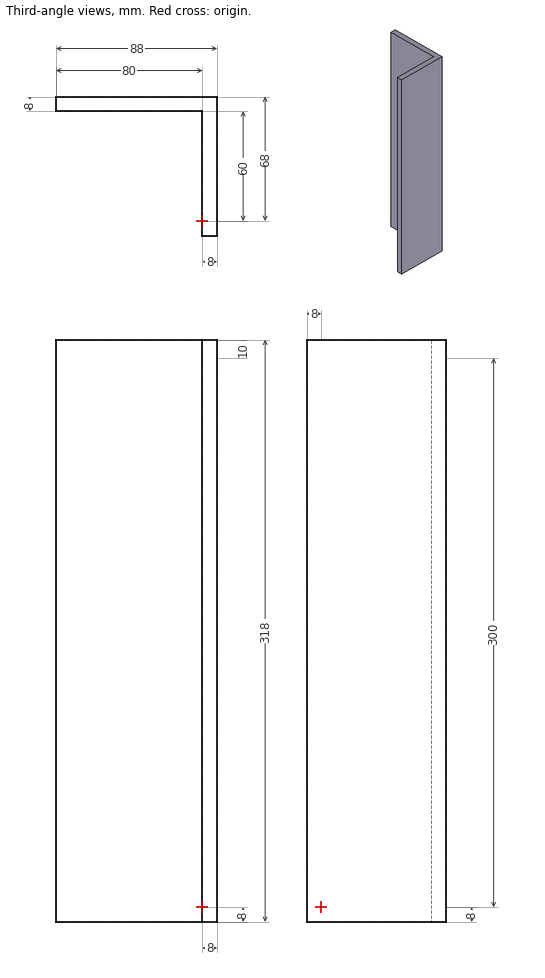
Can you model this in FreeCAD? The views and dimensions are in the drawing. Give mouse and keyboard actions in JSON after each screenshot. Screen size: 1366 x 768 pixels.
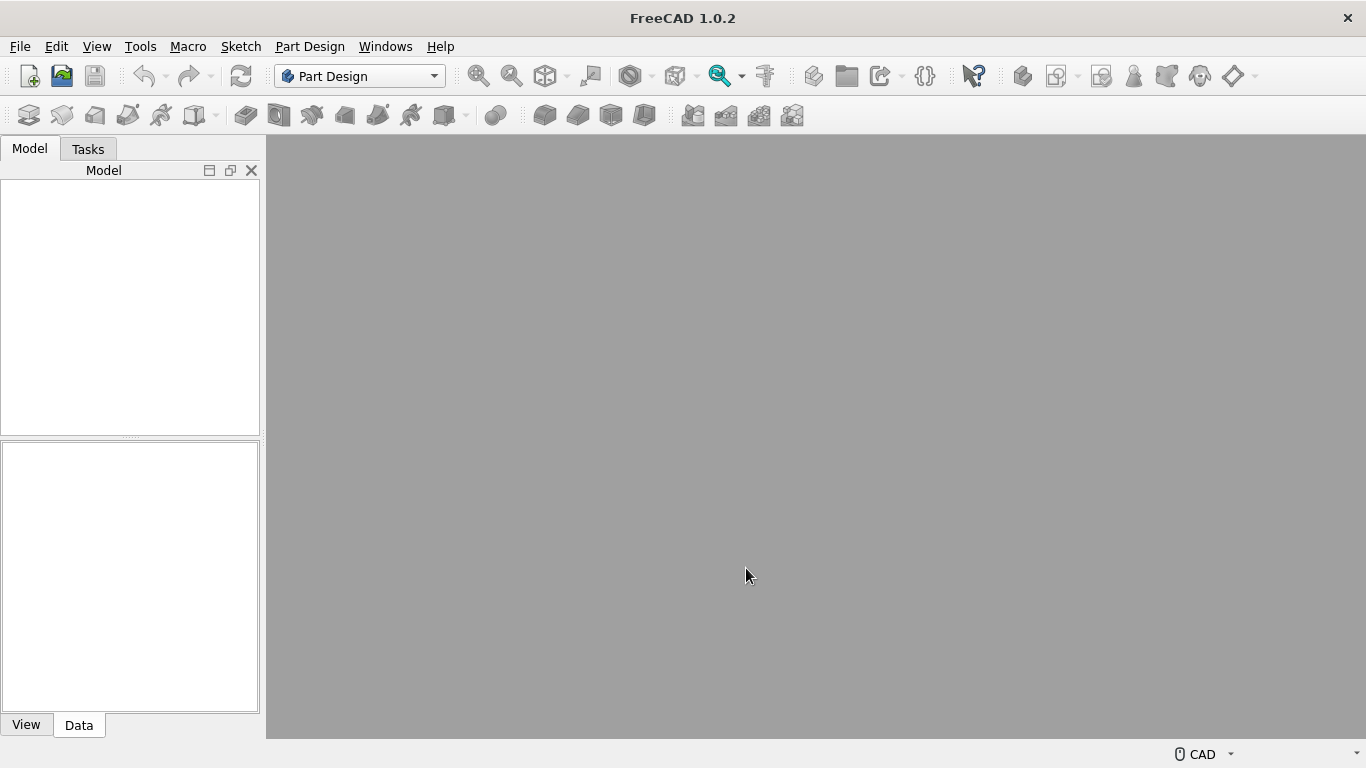
{"action": "left_click", "coordinate": [29, 76]}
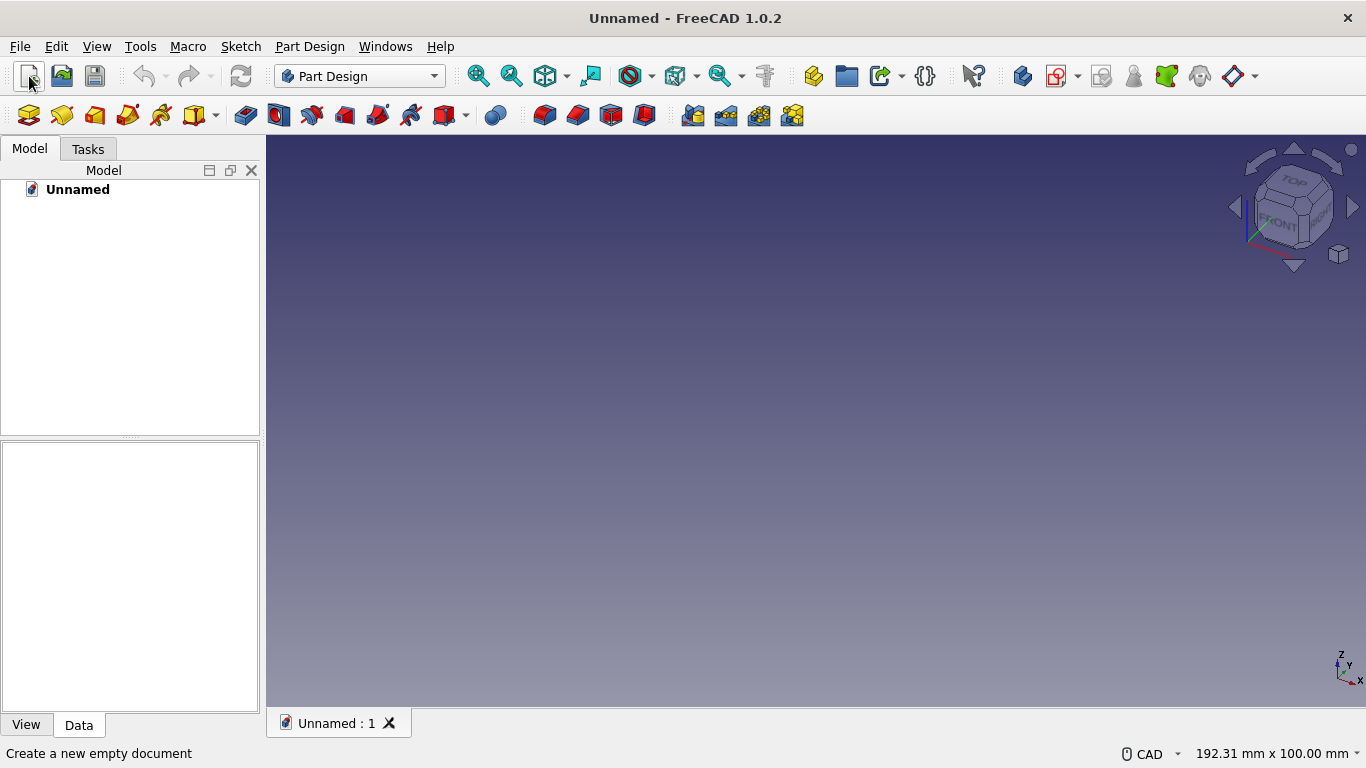
{"action": "left_click", "coordinate": [1056, 76]}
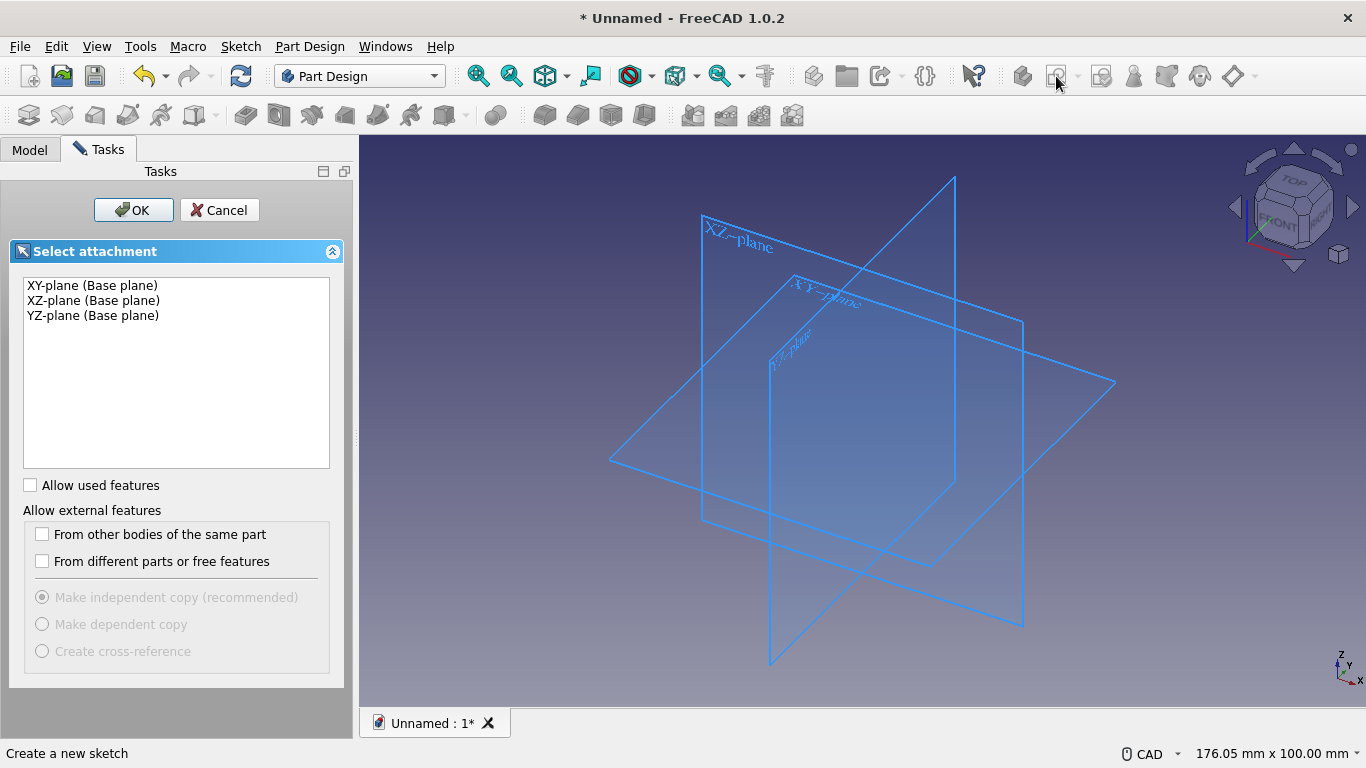
{"action": "left_click", "coordinate": [84, 286]}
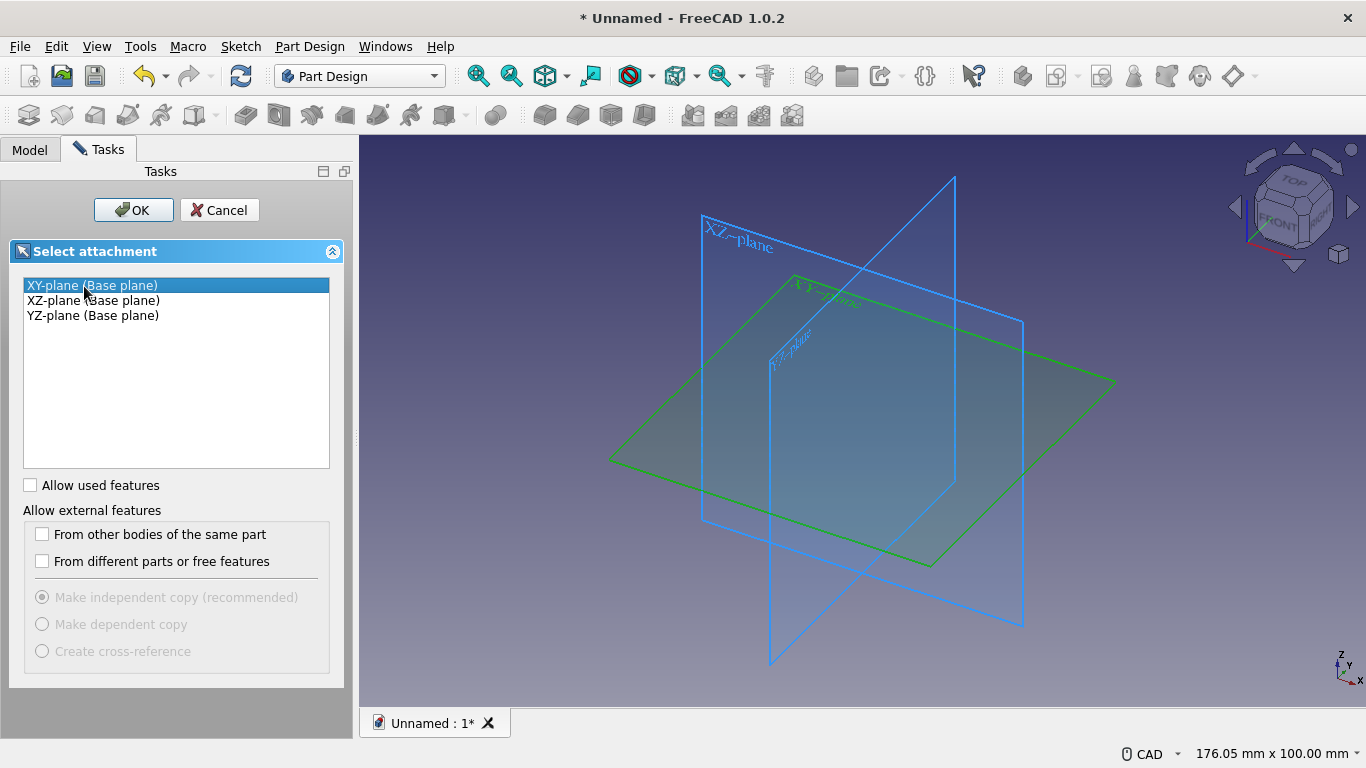
{"action": "left_click", "coordinate": [134, 210]}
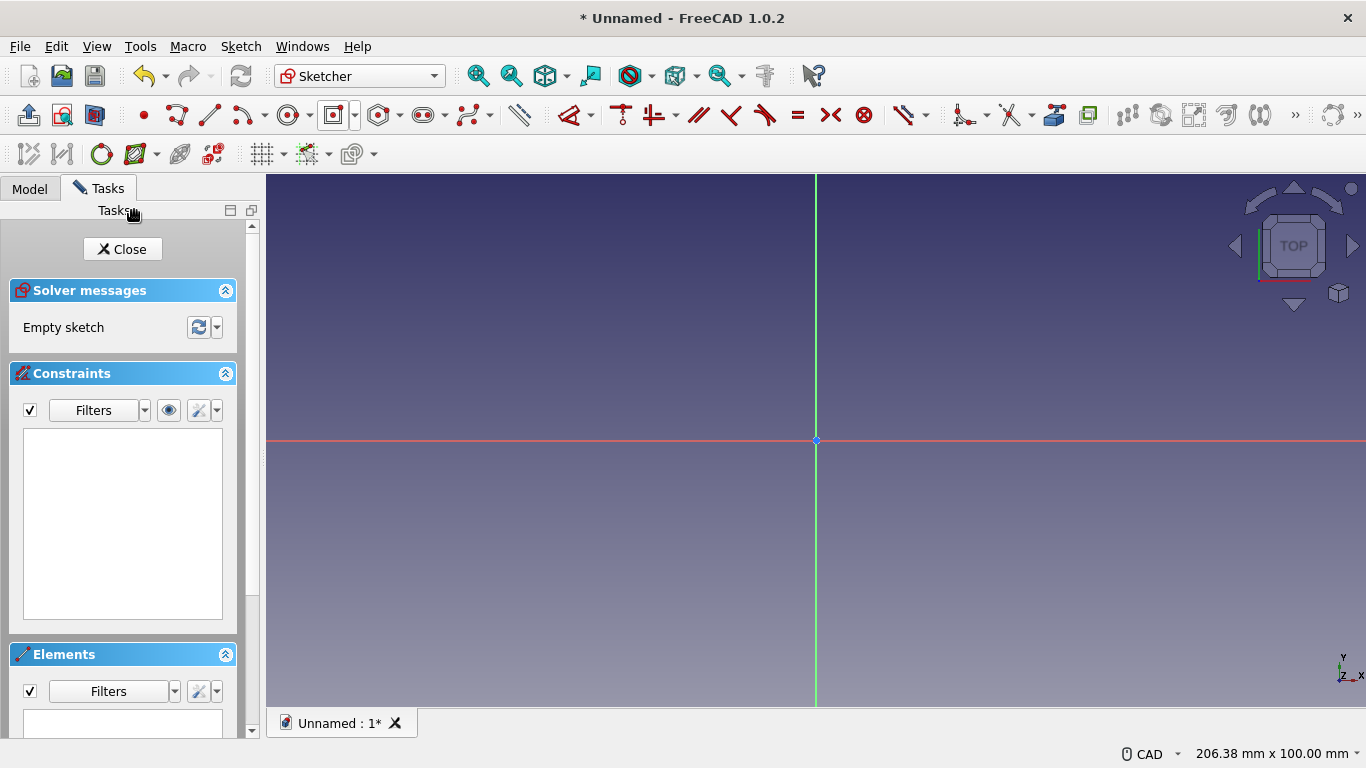
{"action": "scroll", "coordinate": [998, 679], "scroll_direction": "down", "scroll_amount": 2}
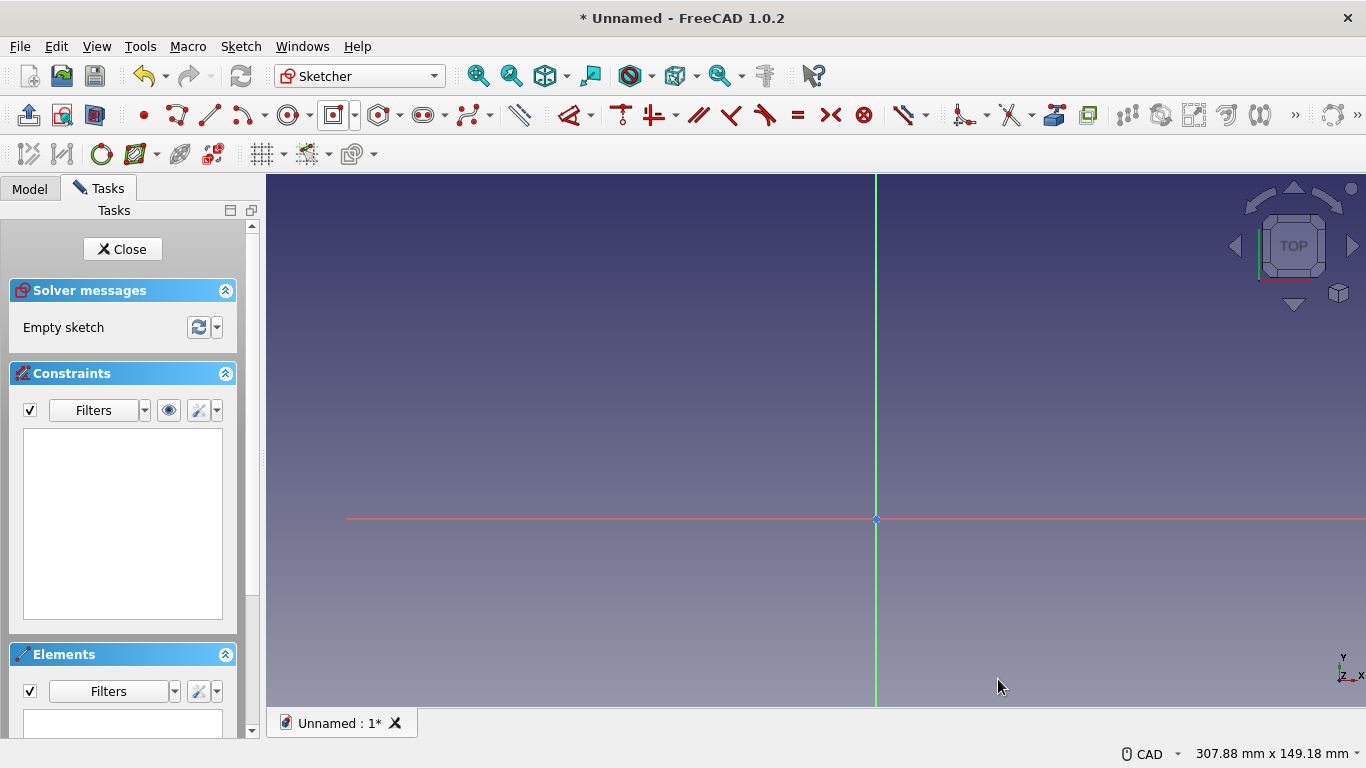
{"action": "scroll", "coordinate": [748, 311], "scroll_direction": "up", "scroll_amount": 2}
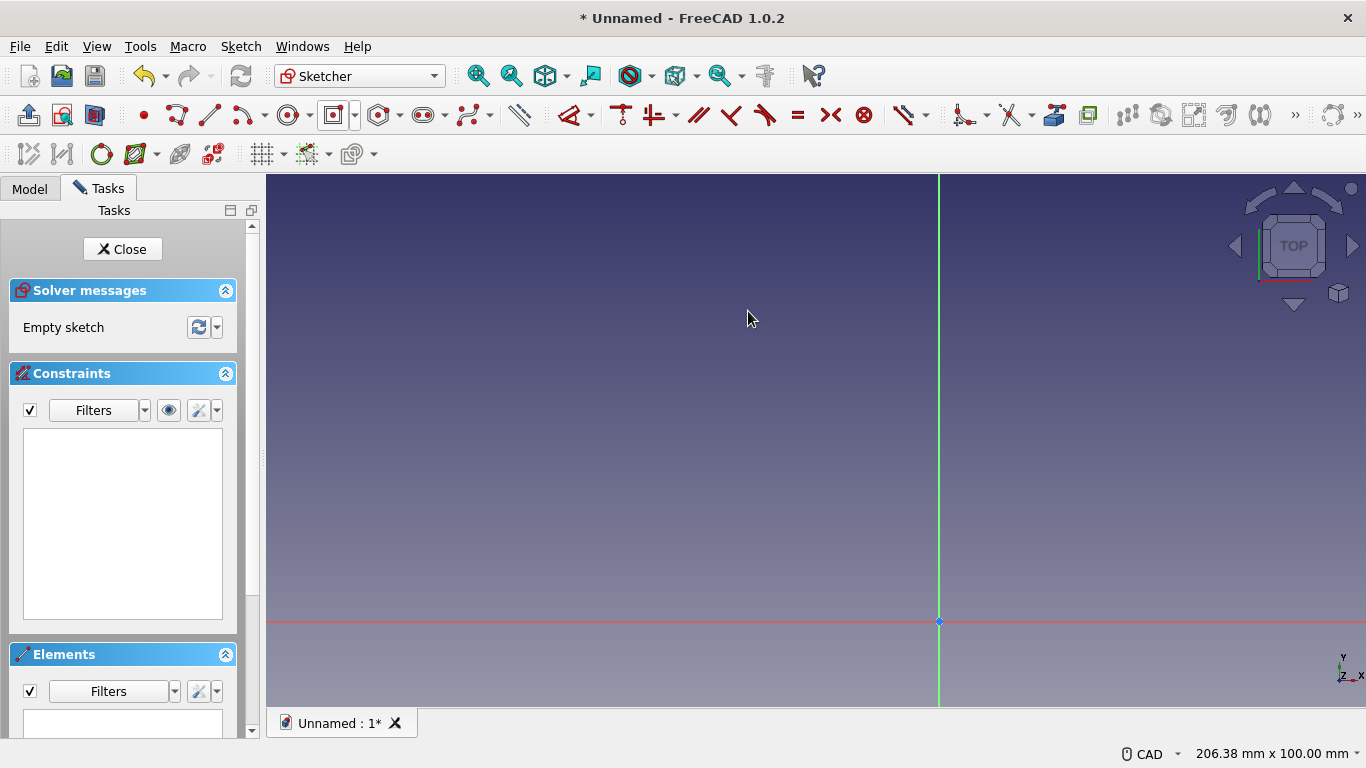
{"action": "key", "text": "g m"}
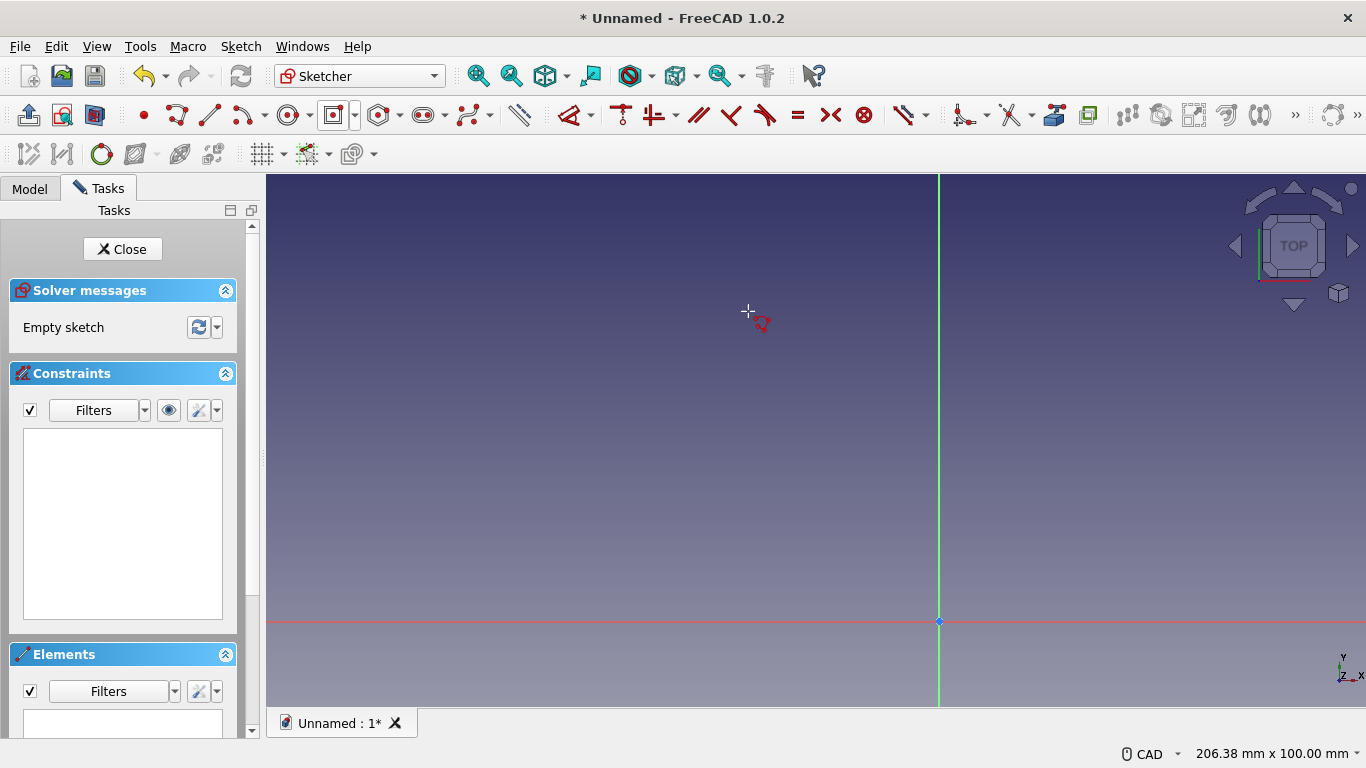
{"action": "left_click", "coordinate": [939, 622]}
{"action": "left_click", "coordinate": [982, 613]}
{"action": "left_click", "coordinate": [982, 259]}
{"action": "left_click", "coordinate": [513, 259]}
{"action": "left_click", "coordinate": [513, 302]}
{"action": "left_click", "coordinate": [930, 302]}
{"action": "left_click", "coordinate": [939, 622]}
{"action": "key", "text": "Escape"}
{"action": "key", "text": "Escape"}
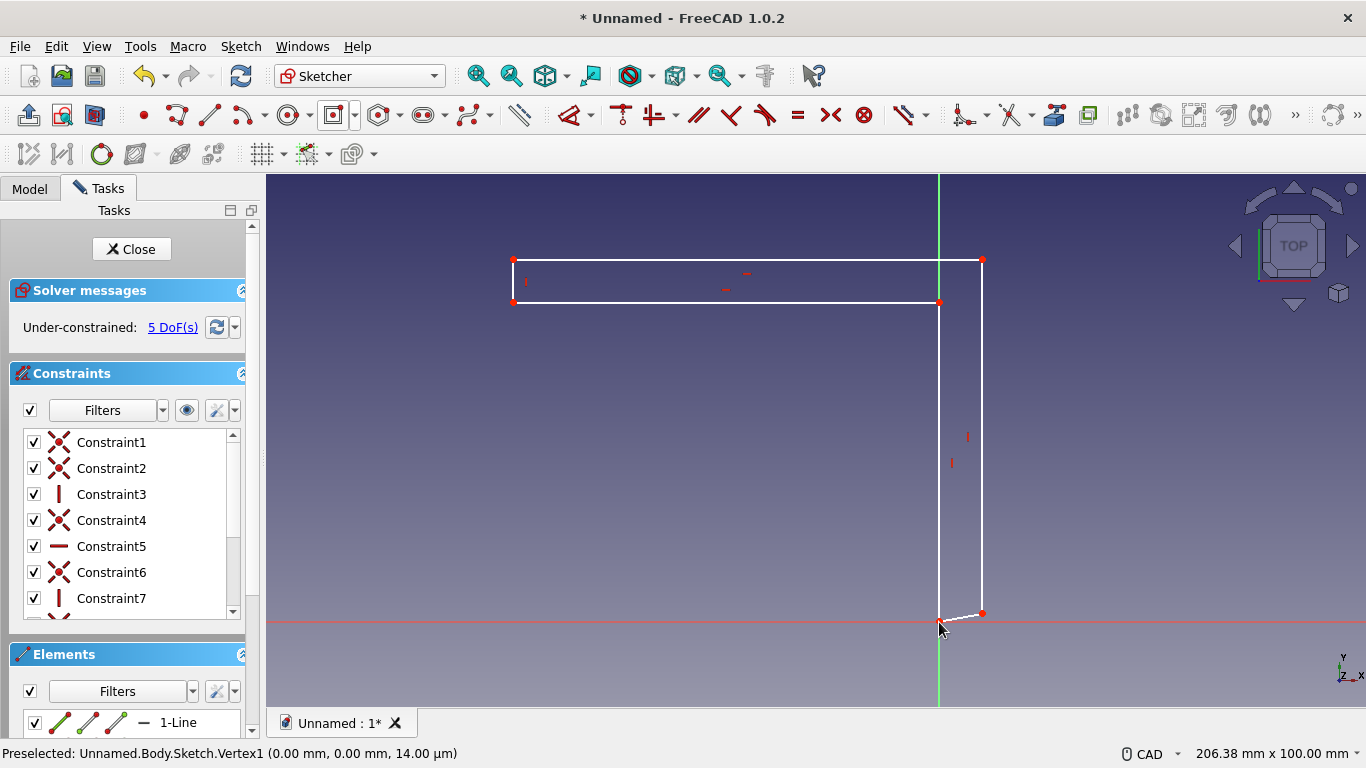
{"action": "left_click", "coordinate": [952, 619]}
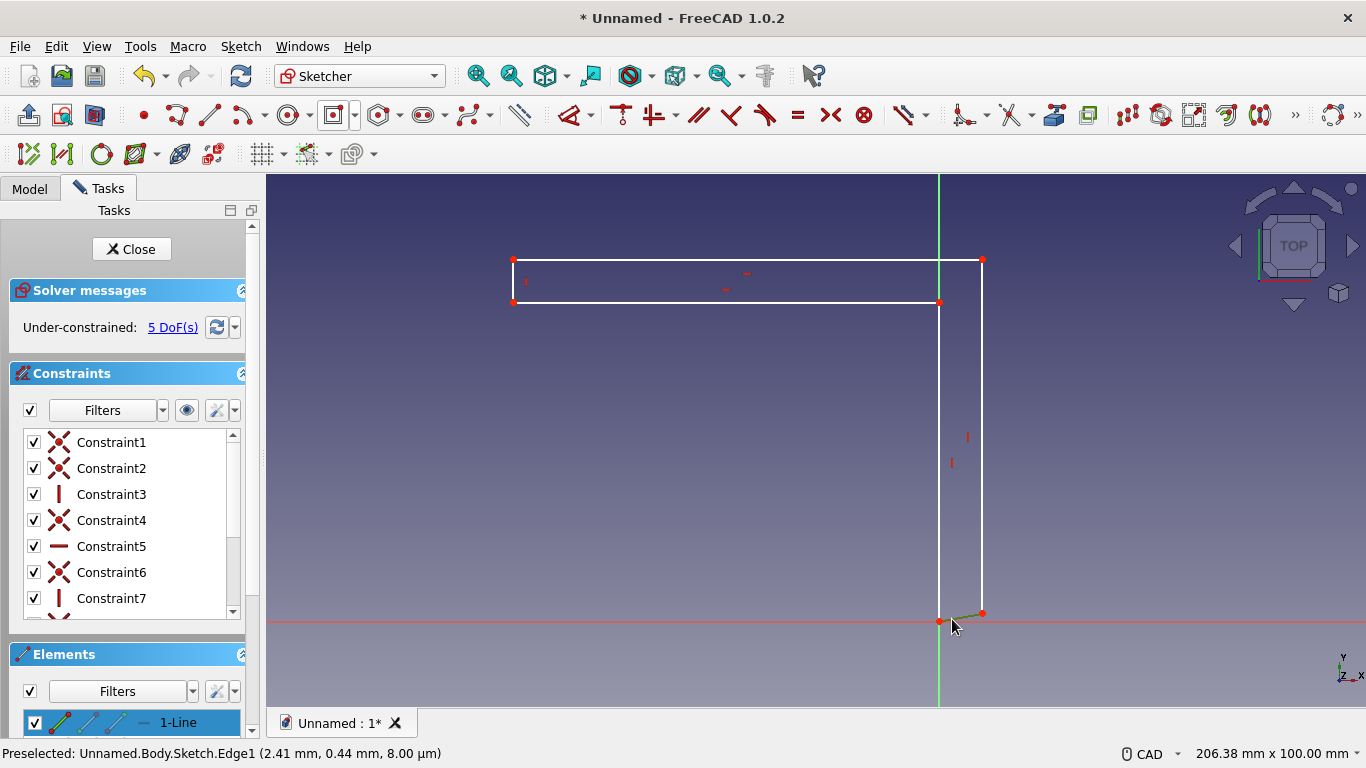
{"action": "key", "text": "h"}